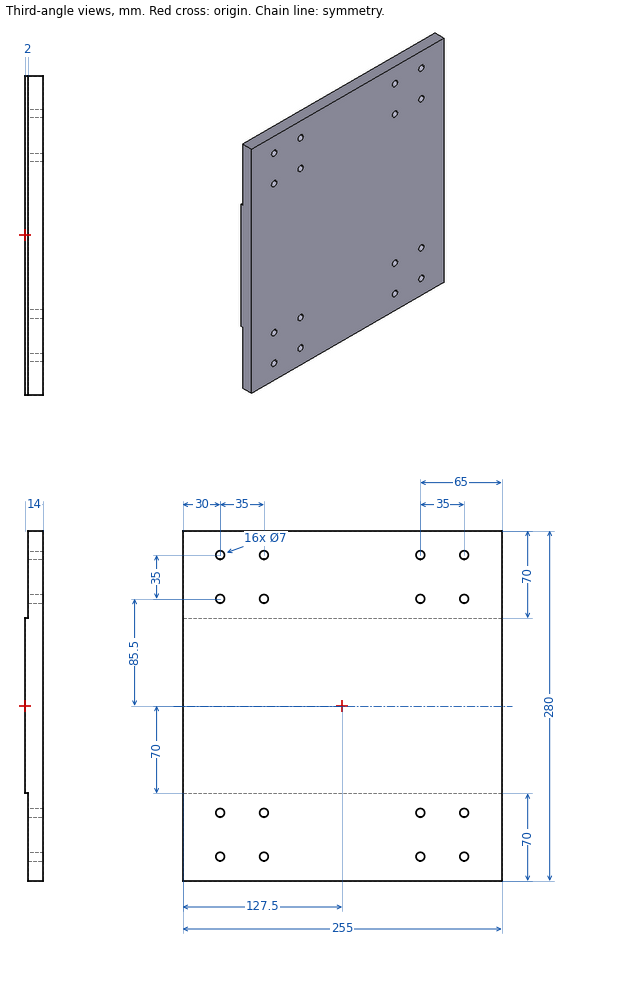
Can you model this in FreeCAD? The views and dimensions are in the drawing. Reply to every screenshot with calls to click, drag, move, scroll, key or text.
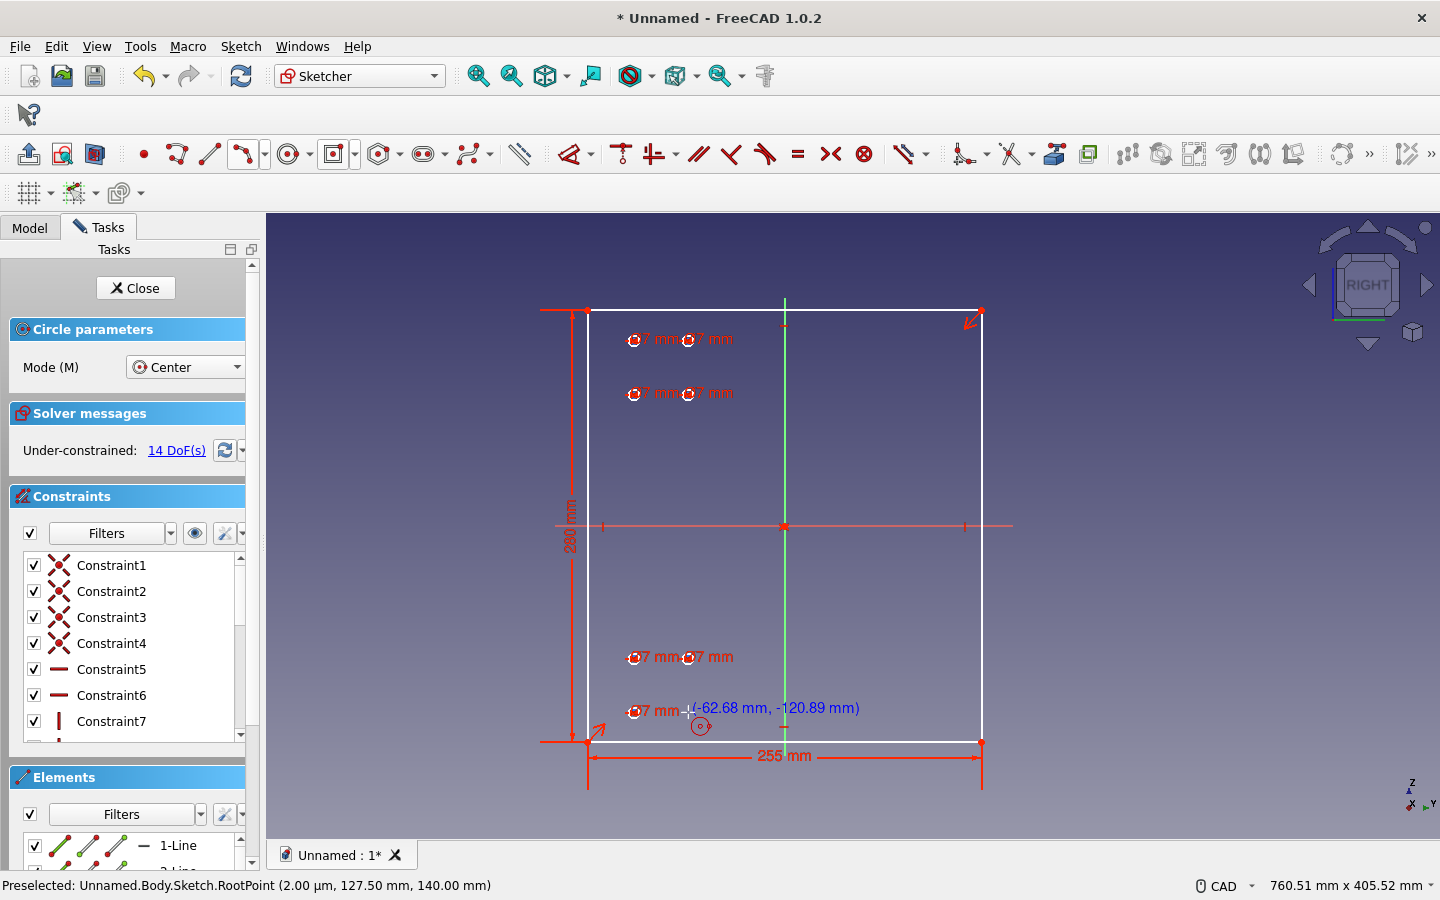
click(688, 712)
move(692, 709)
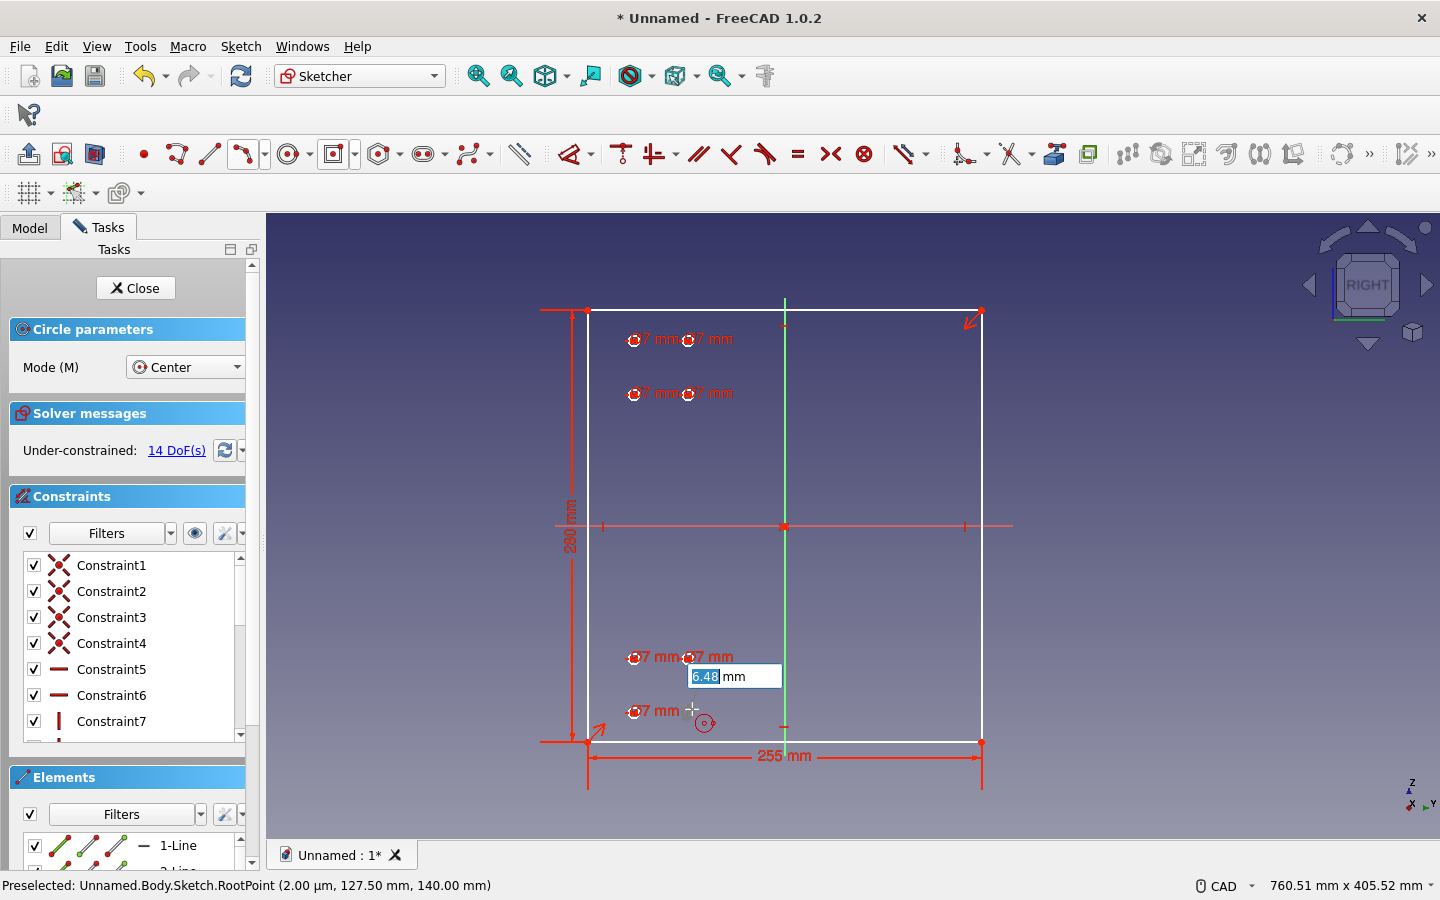
text(7)
key(Return)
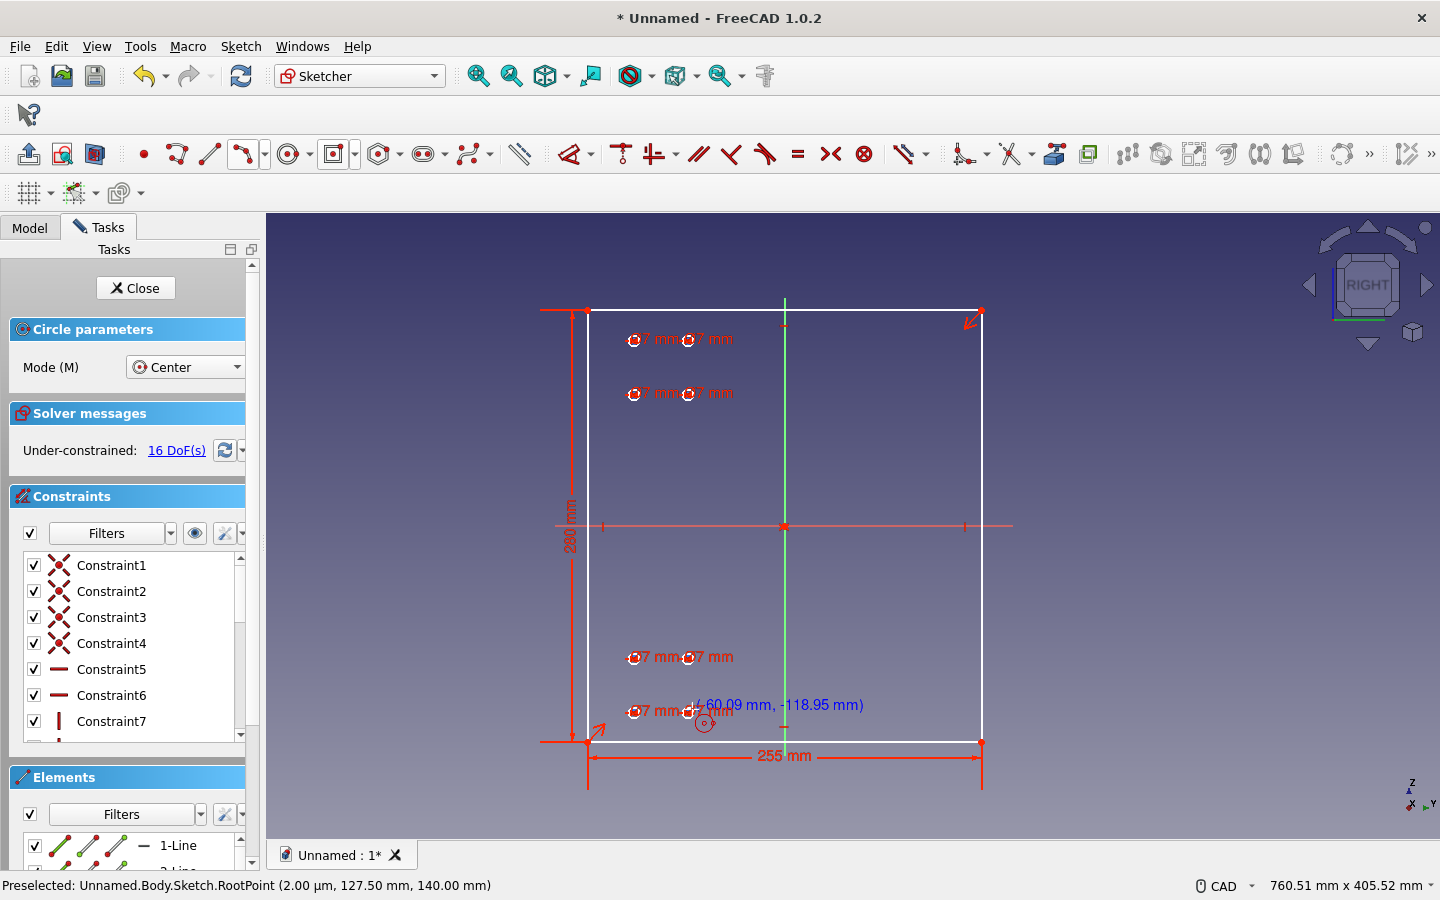
scroll(881, 340, up, 8)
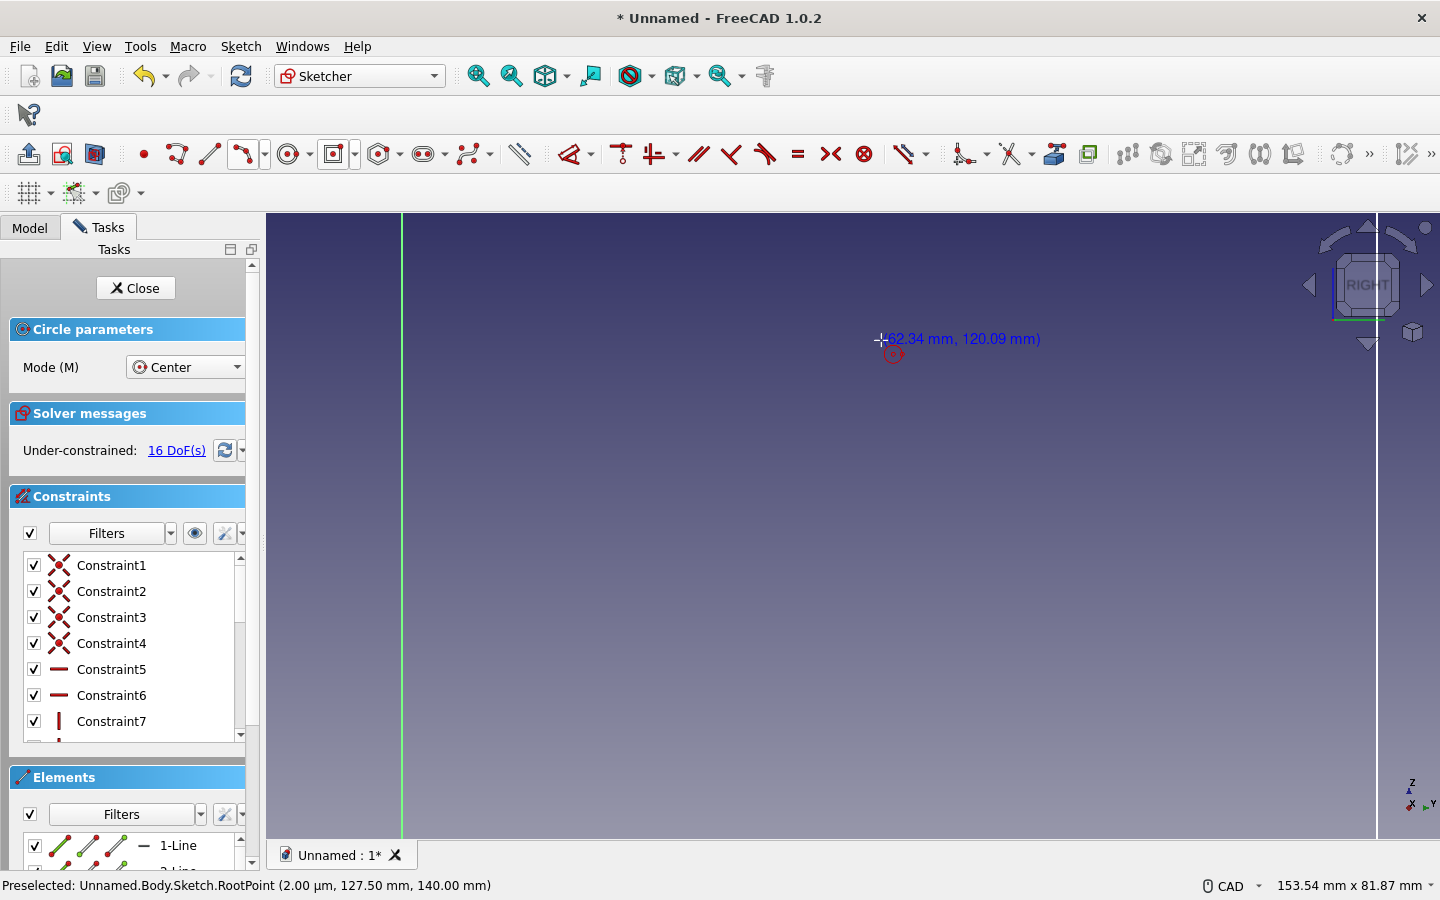
scroll(881, 340, down, 8)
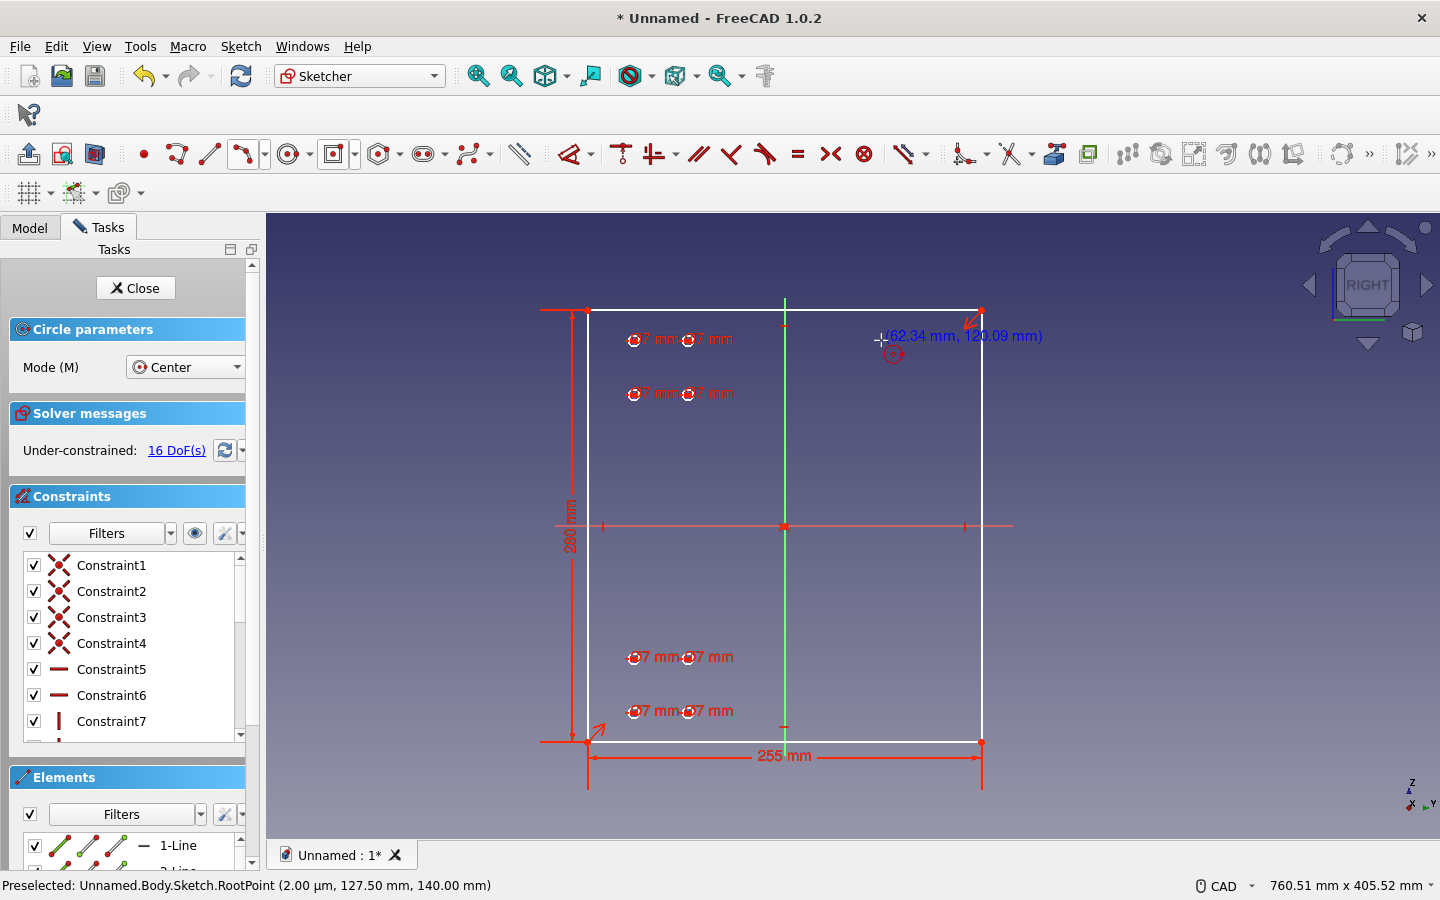
click(881, 340)
move(885, 337)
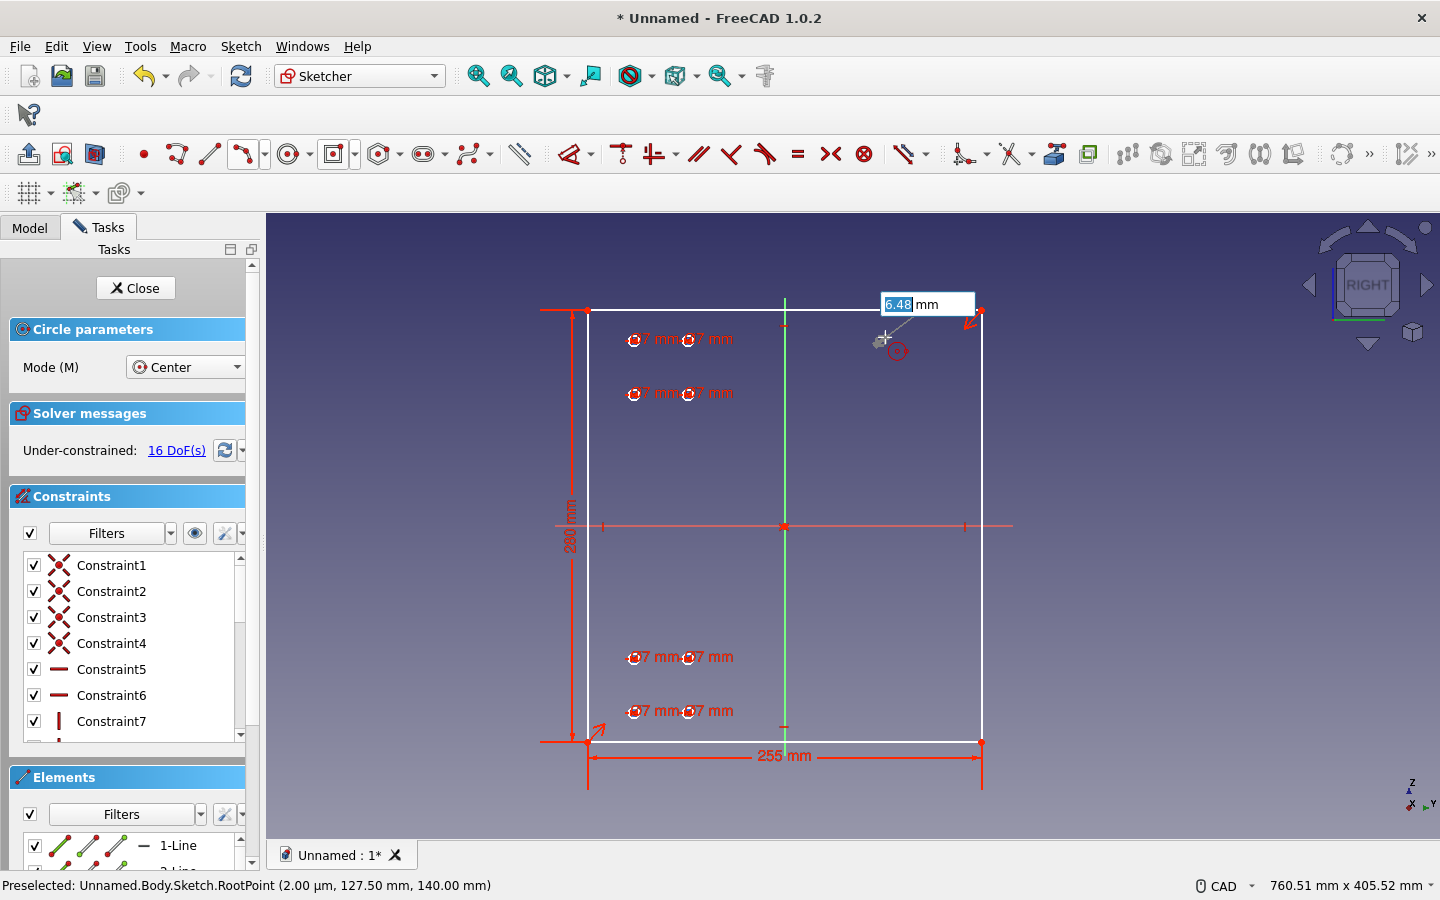
text(7)
key(Return)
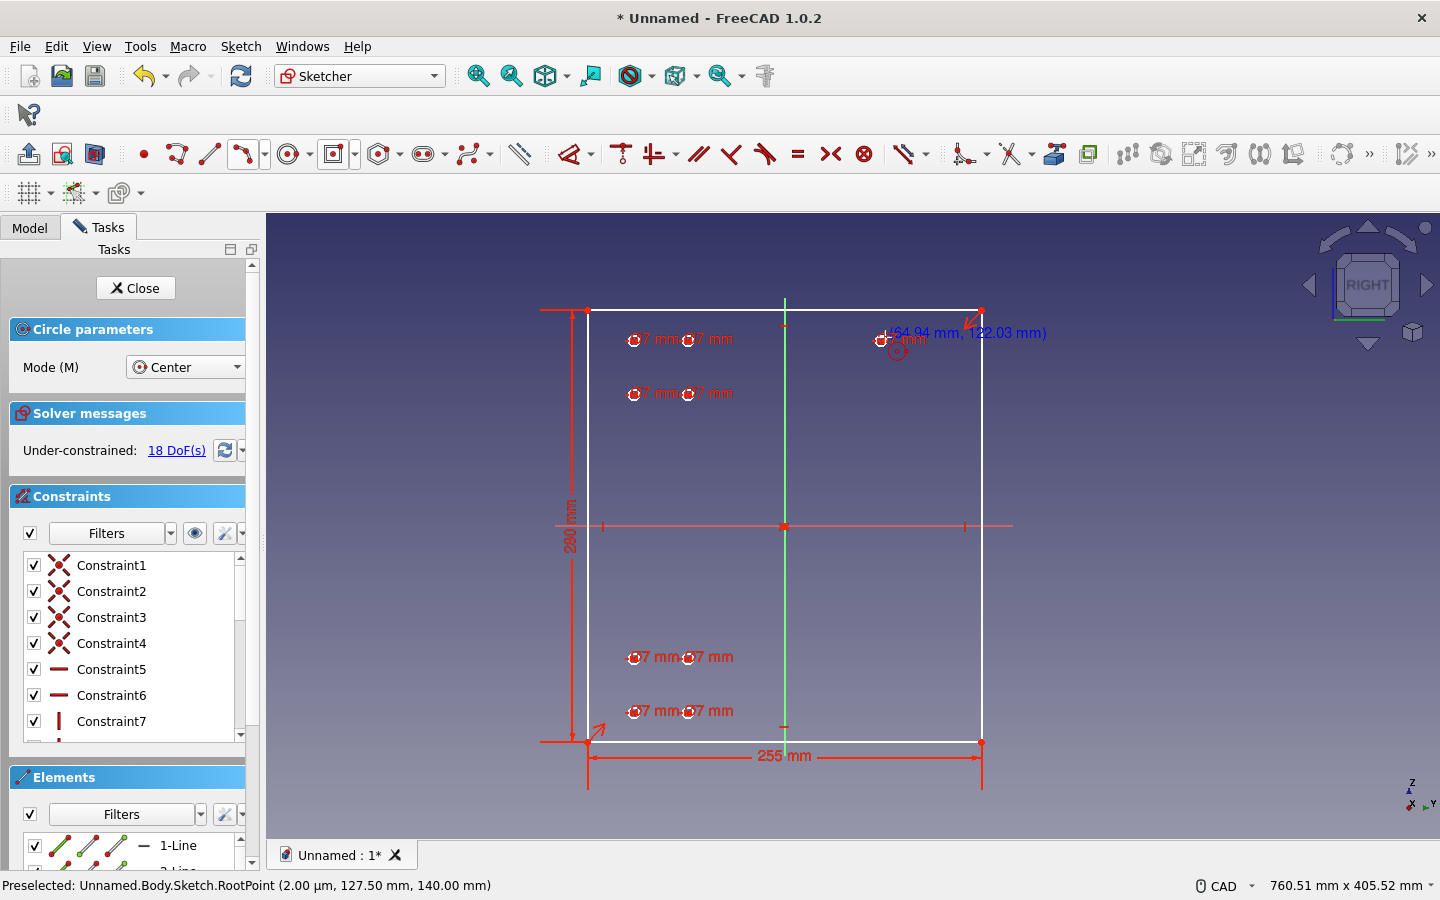
scroll(881, 394, up, 8)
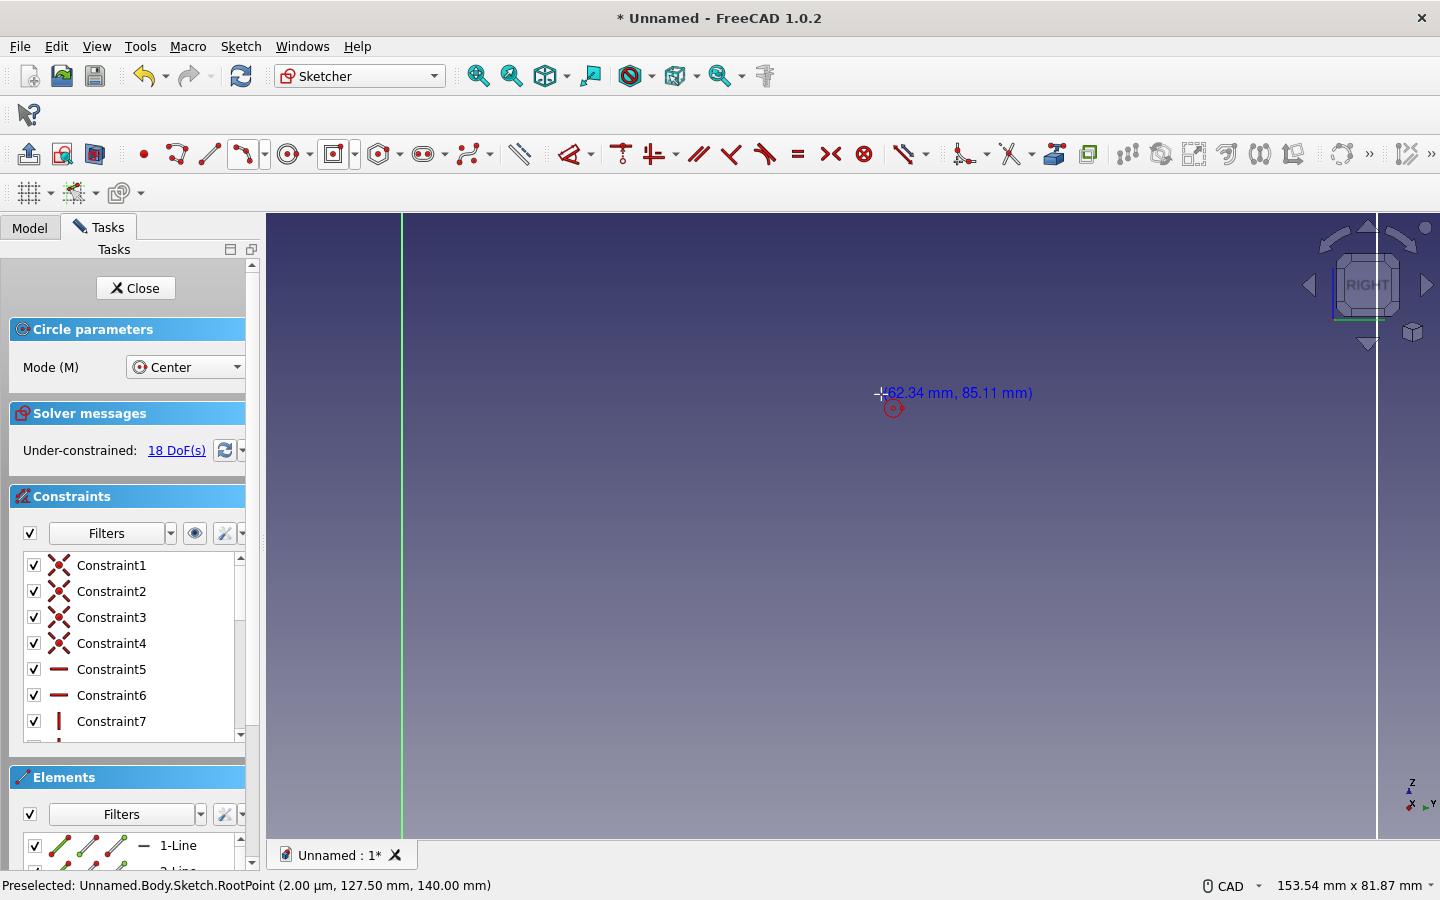
scroll(881, 394, down, 8)